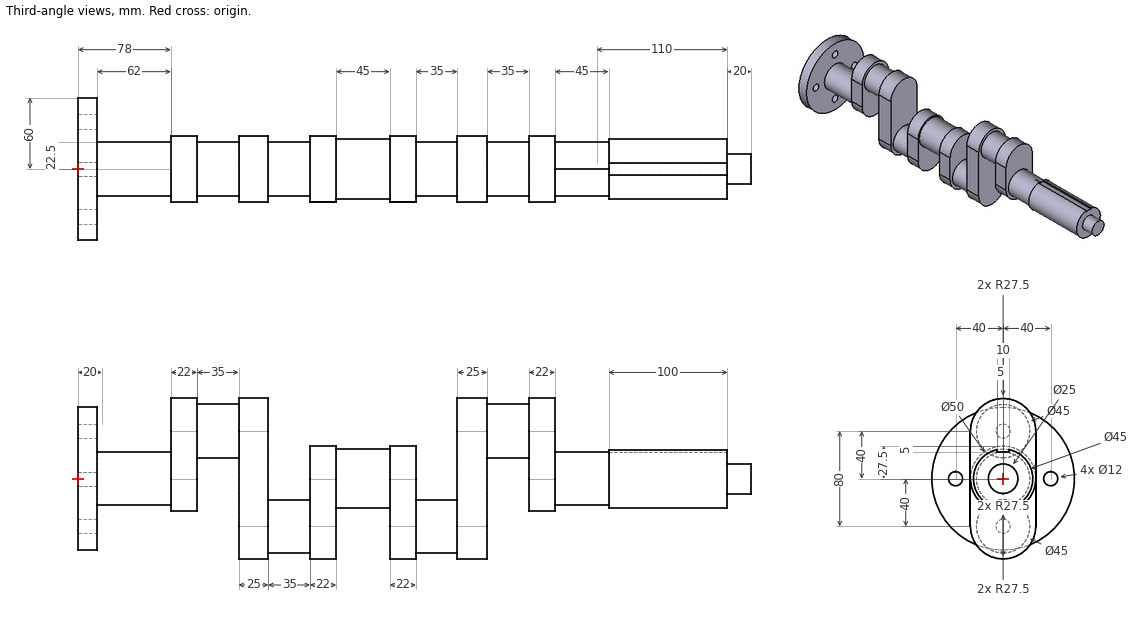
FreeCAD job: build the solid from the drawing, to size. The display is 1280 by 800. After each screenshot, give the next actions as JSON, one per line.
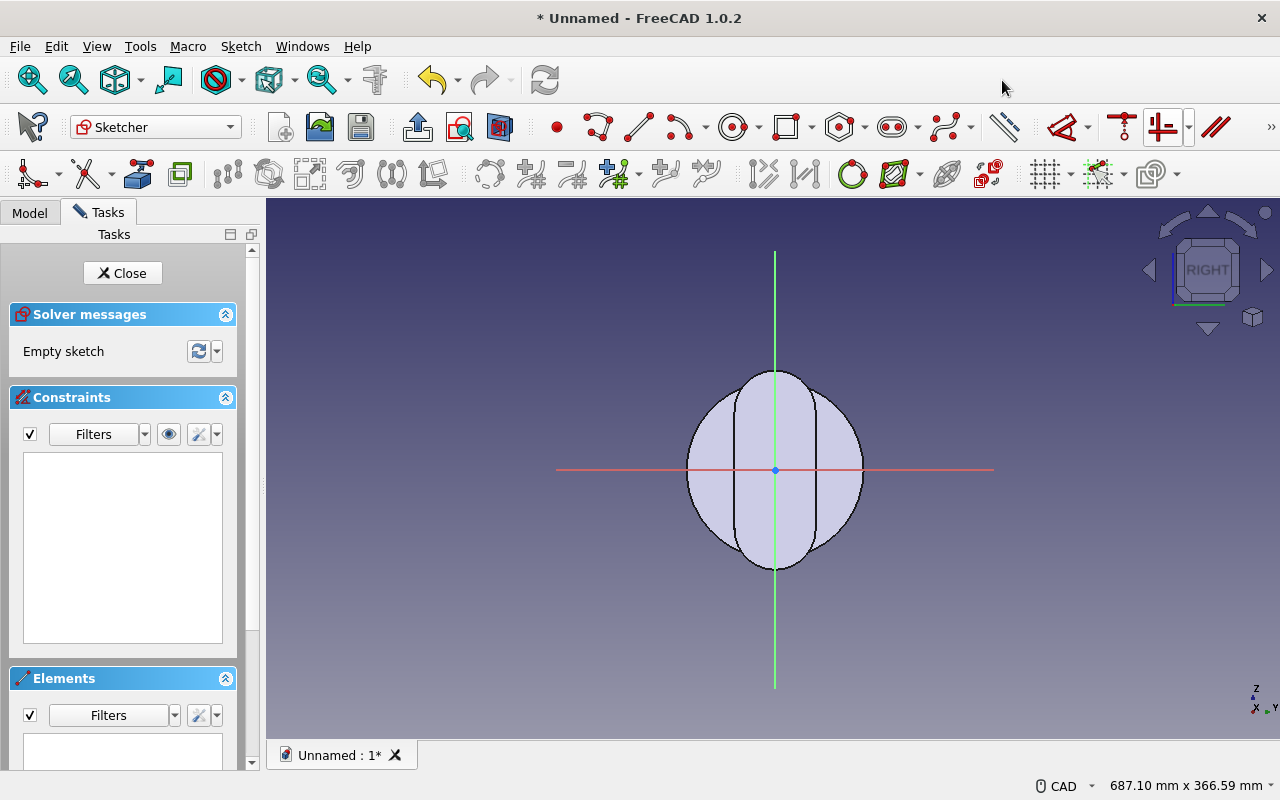
{"action": "scroll", "coordinate": [798, 410], "scroll_direction": "up", "scroll_amount": 7}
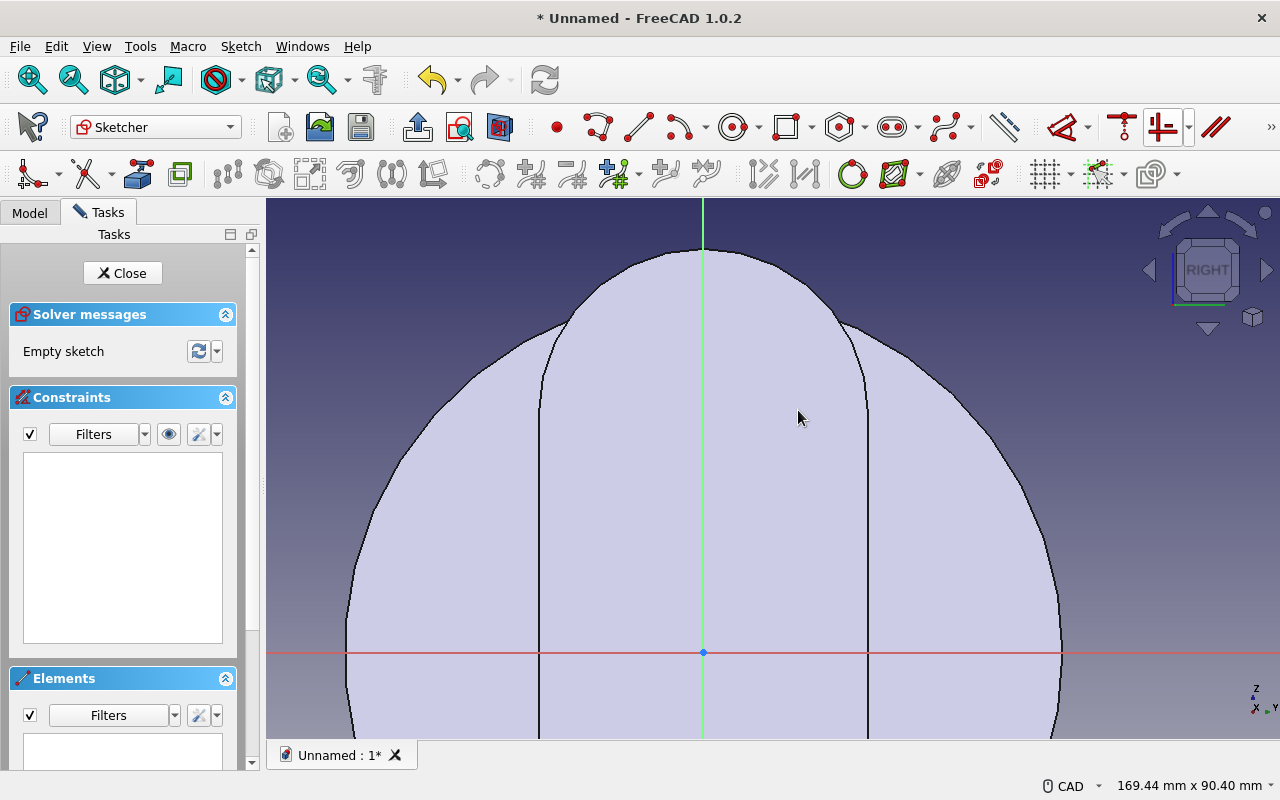
{"action": "key", "text": "g c"}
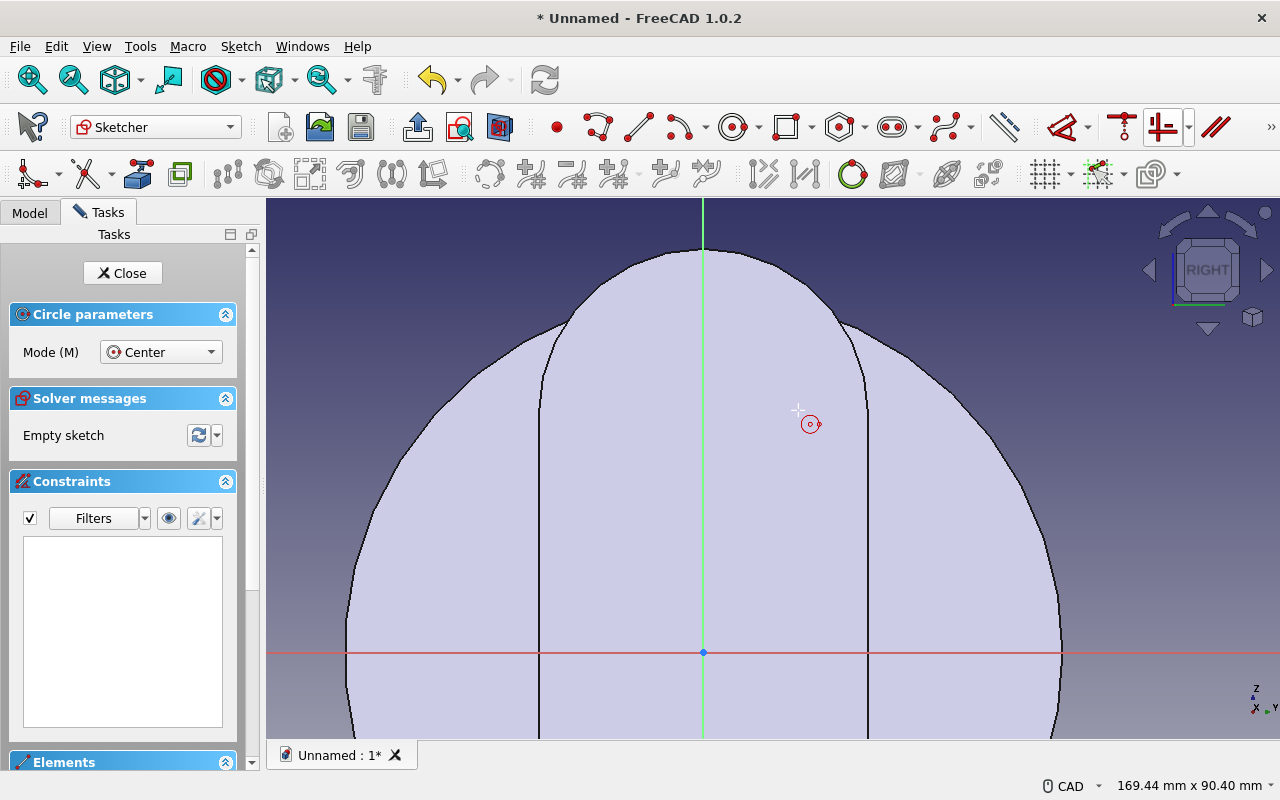
{"action": "left_click", "coordinate": [703, 413]}
{"action": "left_click", "coordinate": [799, 318]}
{"action": "key", "text": "Escape"}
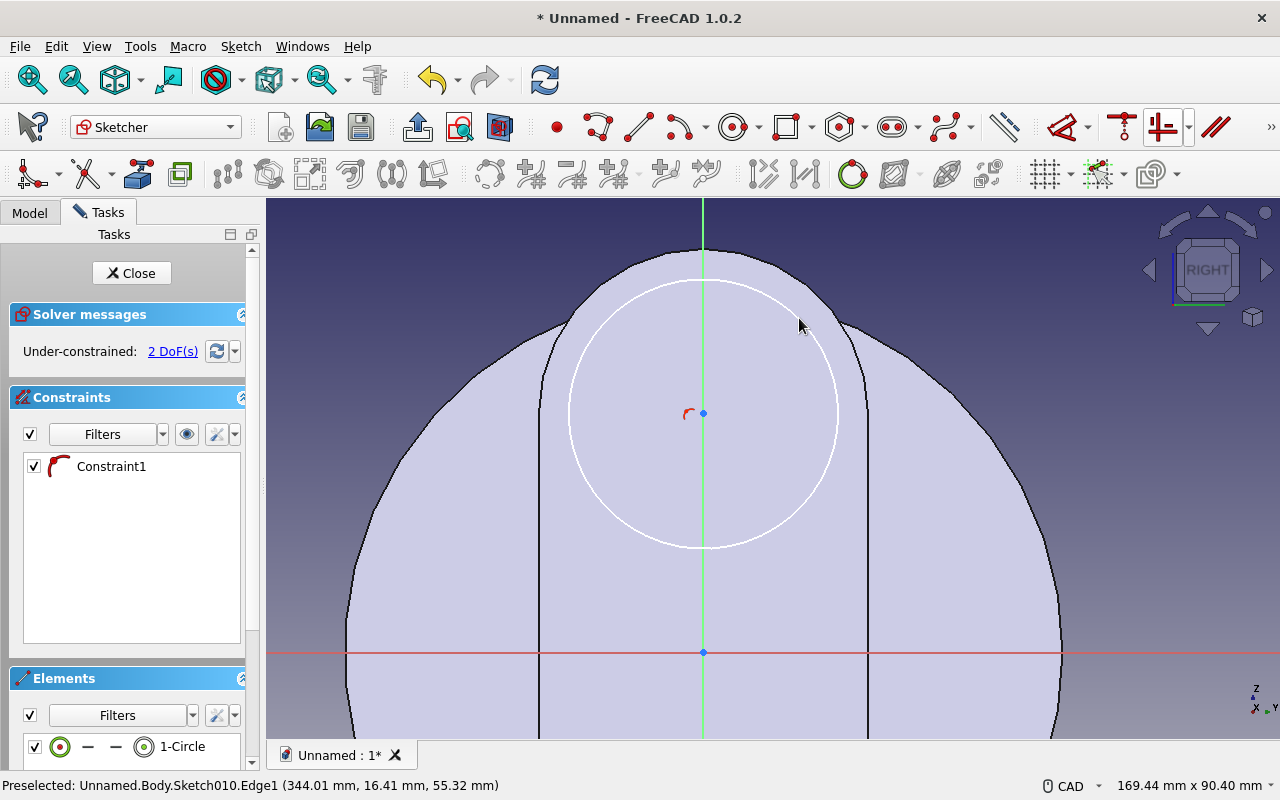
{"action": "left_click", "coordinate": [1062, 128]}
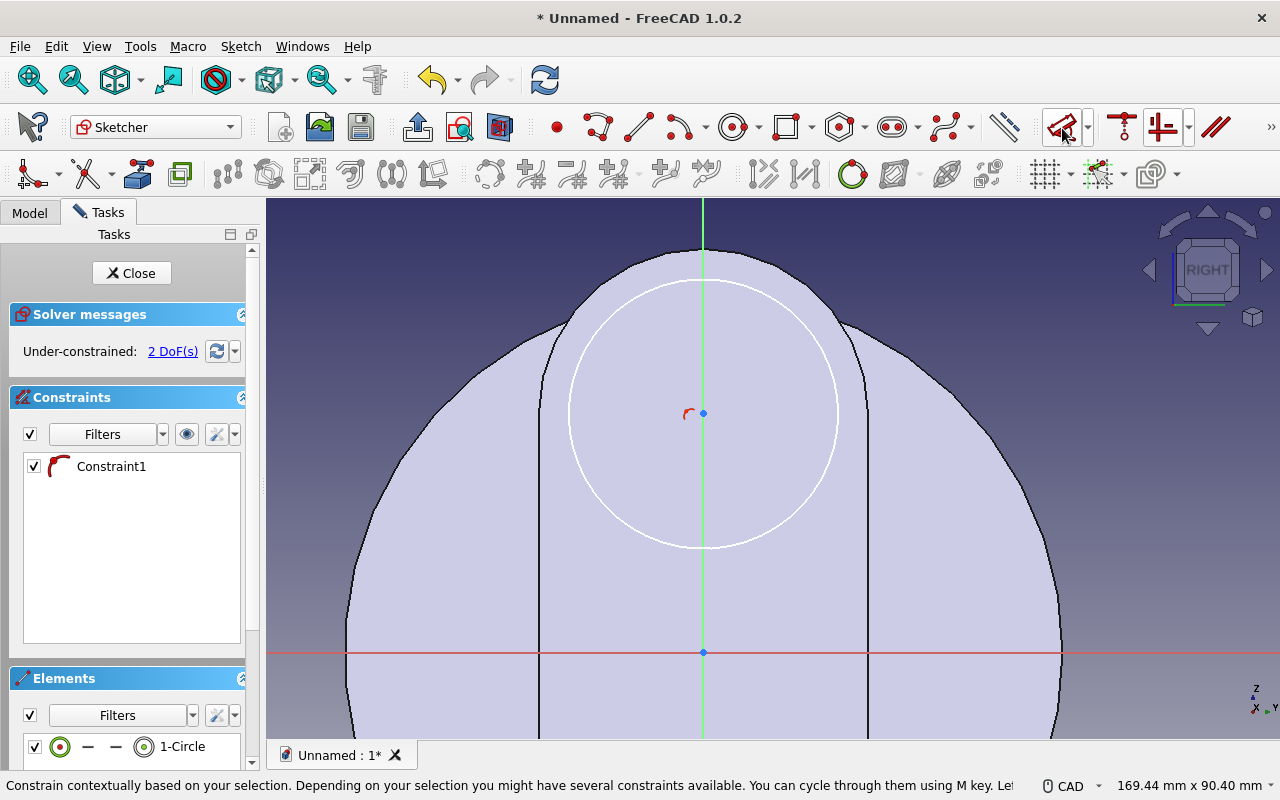
{"action": "left_click", "coordinate": [798, 318]}
{"action": "left_click", "coordinate": [820, 295]}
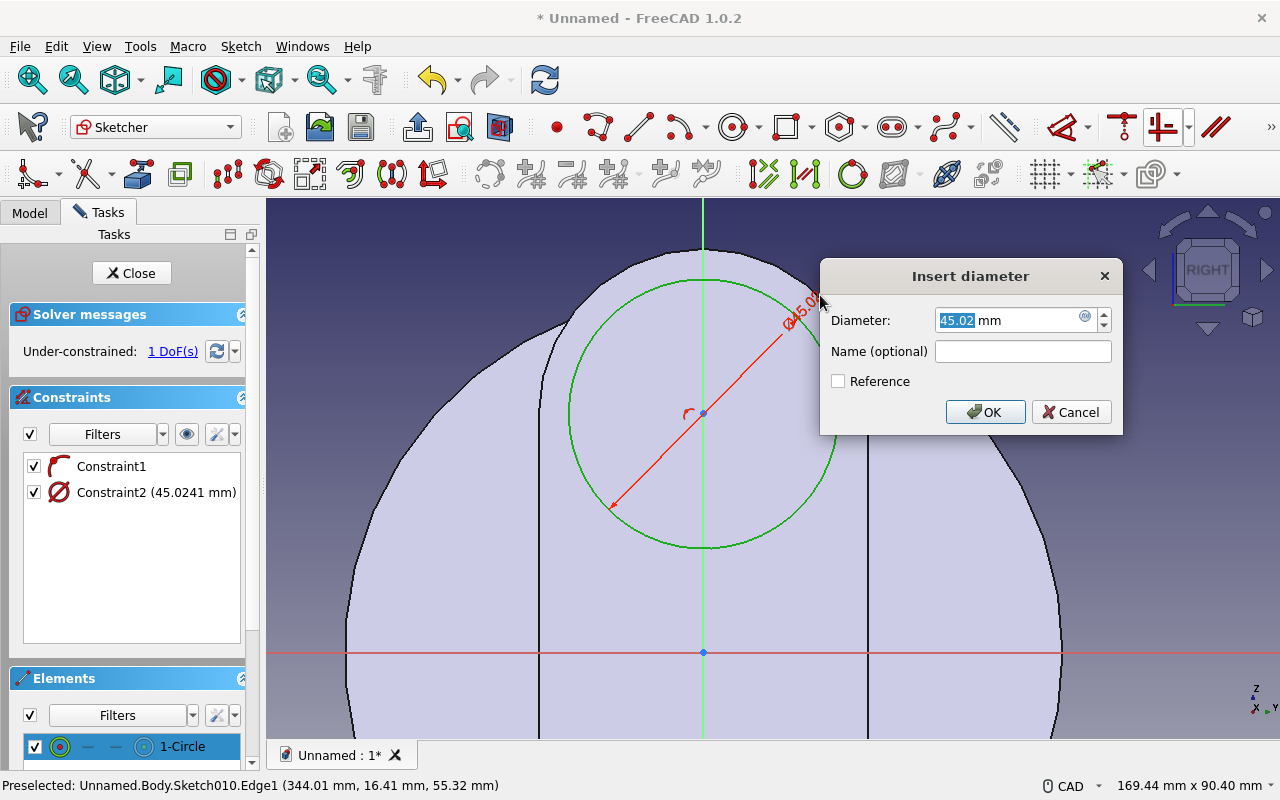
{"action": "type", "text": "45"}
{"action": "key", "text": "Return"}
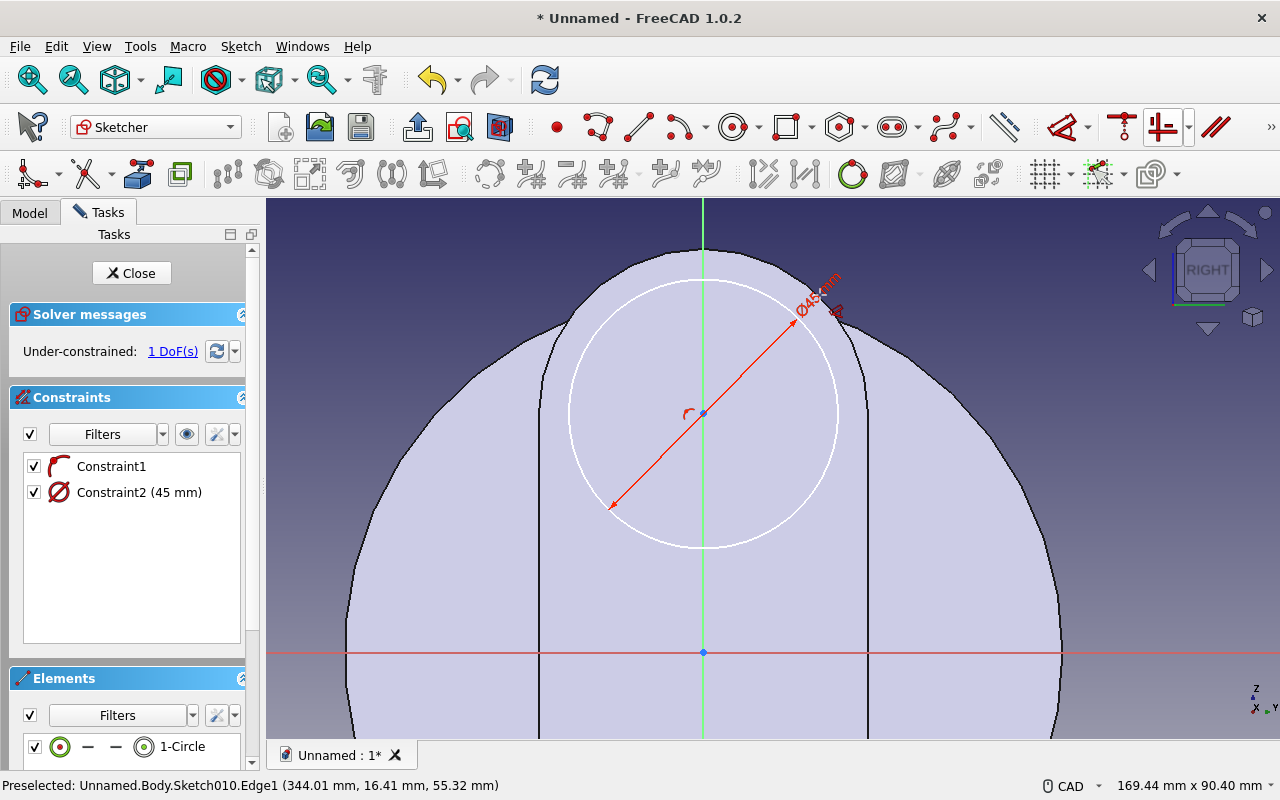
{"action": "left_click", "coordinate": [703, 414]}
{"action": "left_click", "coordinate": [737, 478]}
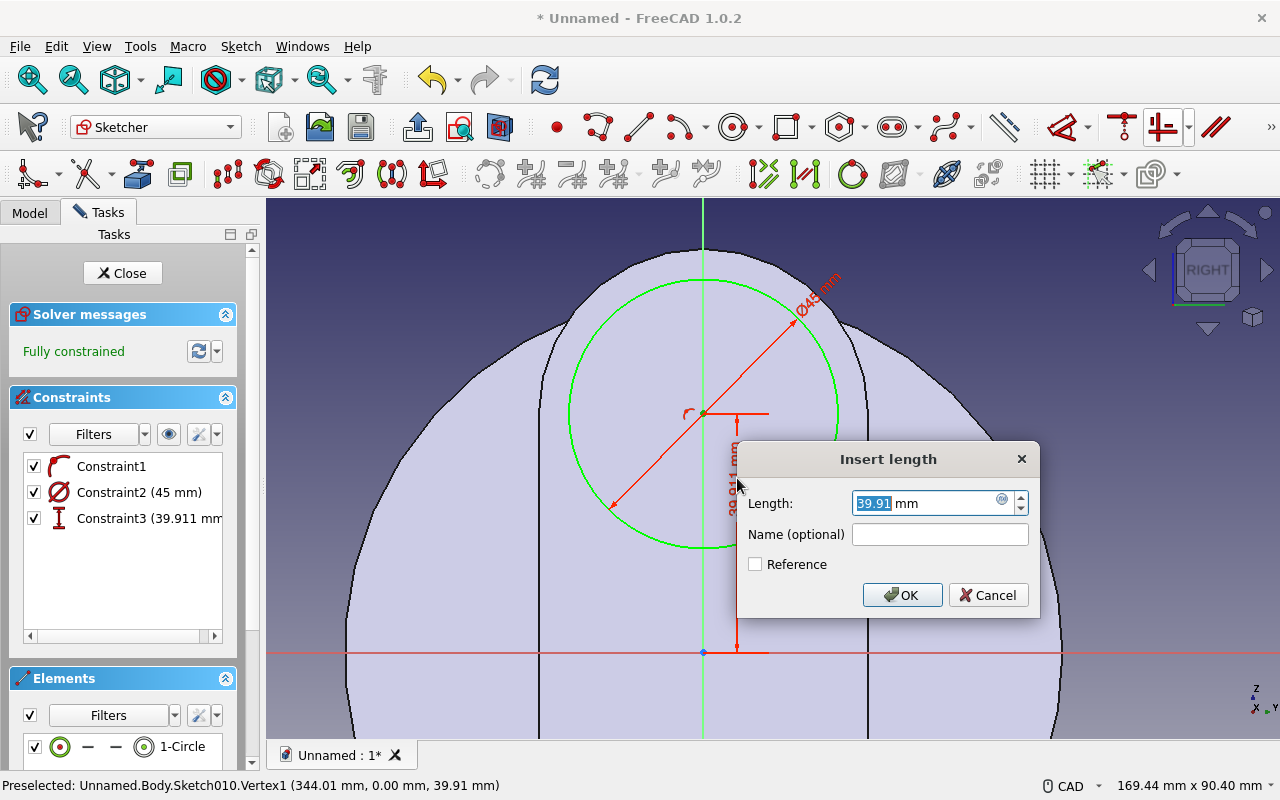
{"action": "type", "text": "40"}
{"action": "key", "text": "Return"}
{"action": "key", "text": "Escape"}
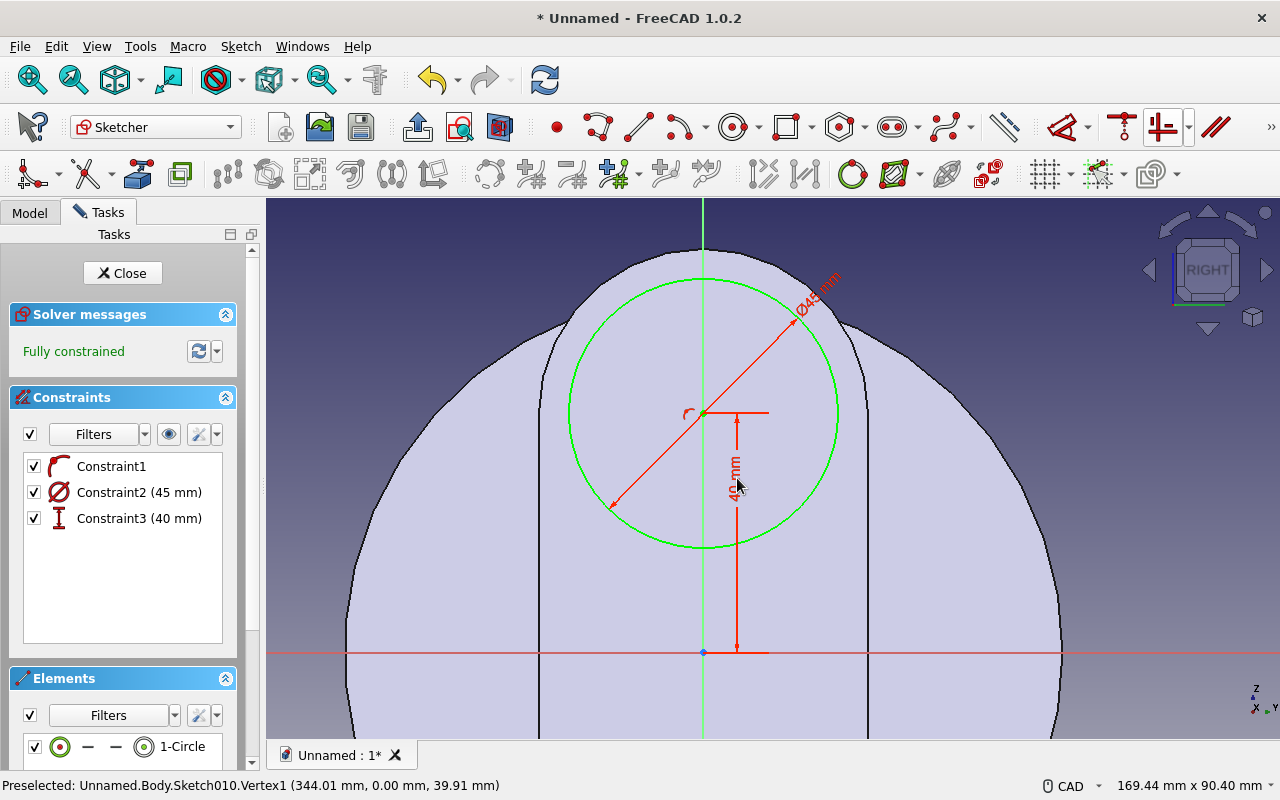
{"action": "left_click", "coordinate": [123, 273]}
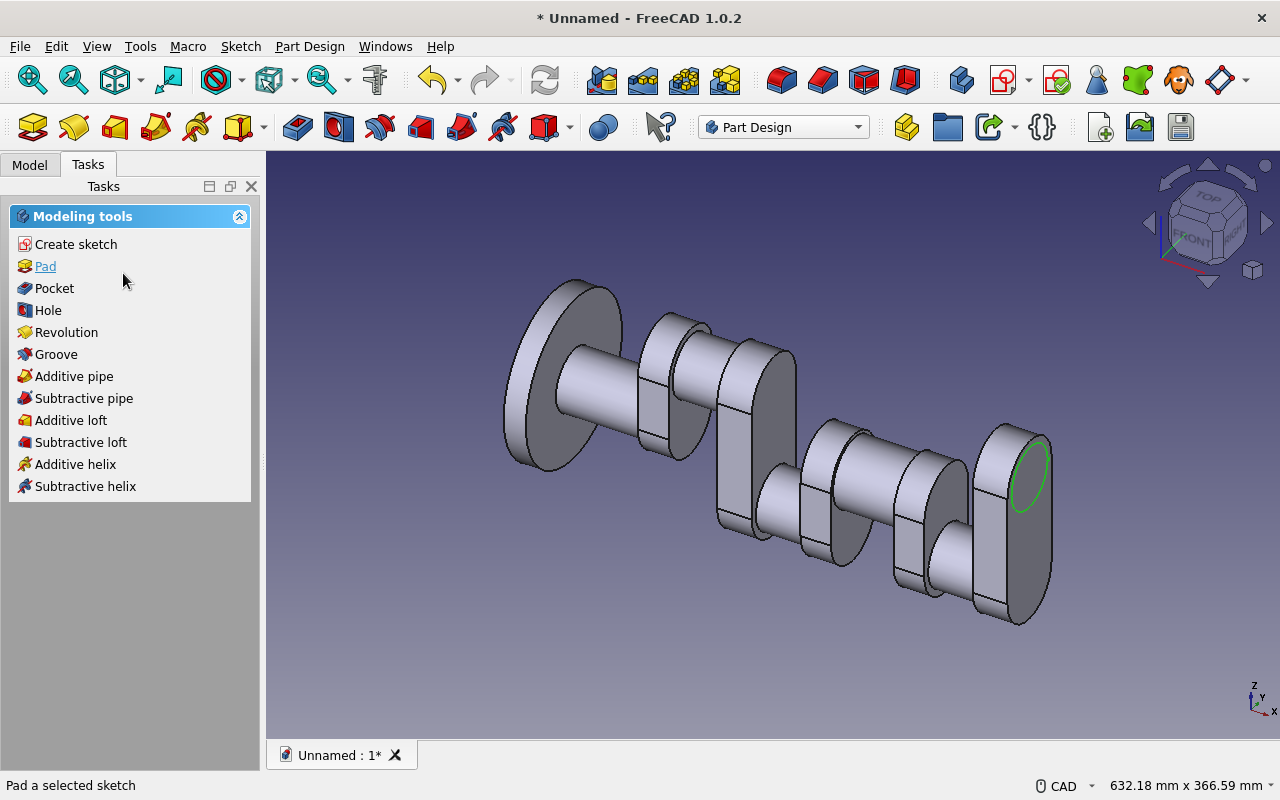
{"action": "left_click", "coordinate": [33, 128]}